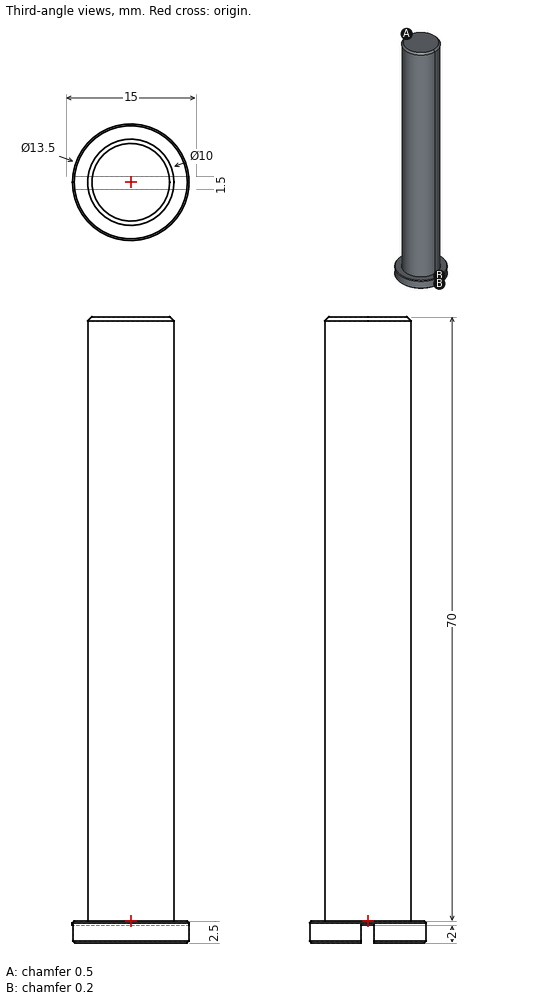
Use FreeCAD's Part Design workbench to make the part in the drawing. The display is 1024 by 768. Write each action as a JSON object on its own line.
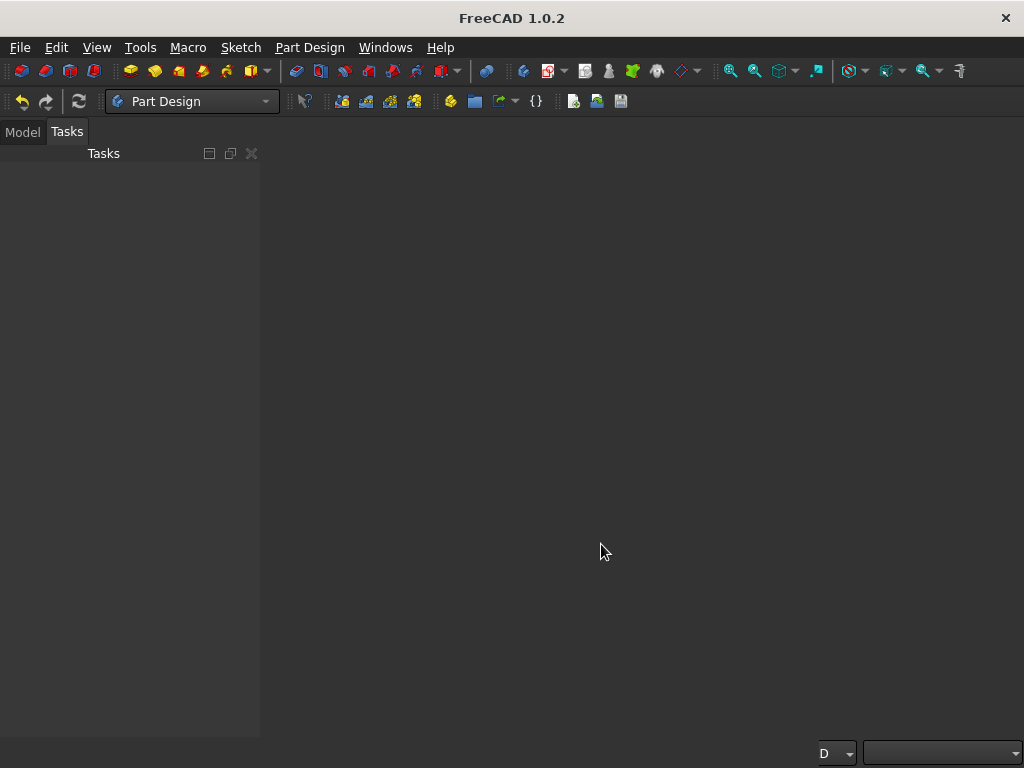
{"action": "left_click", "coordinate": [574, 102]}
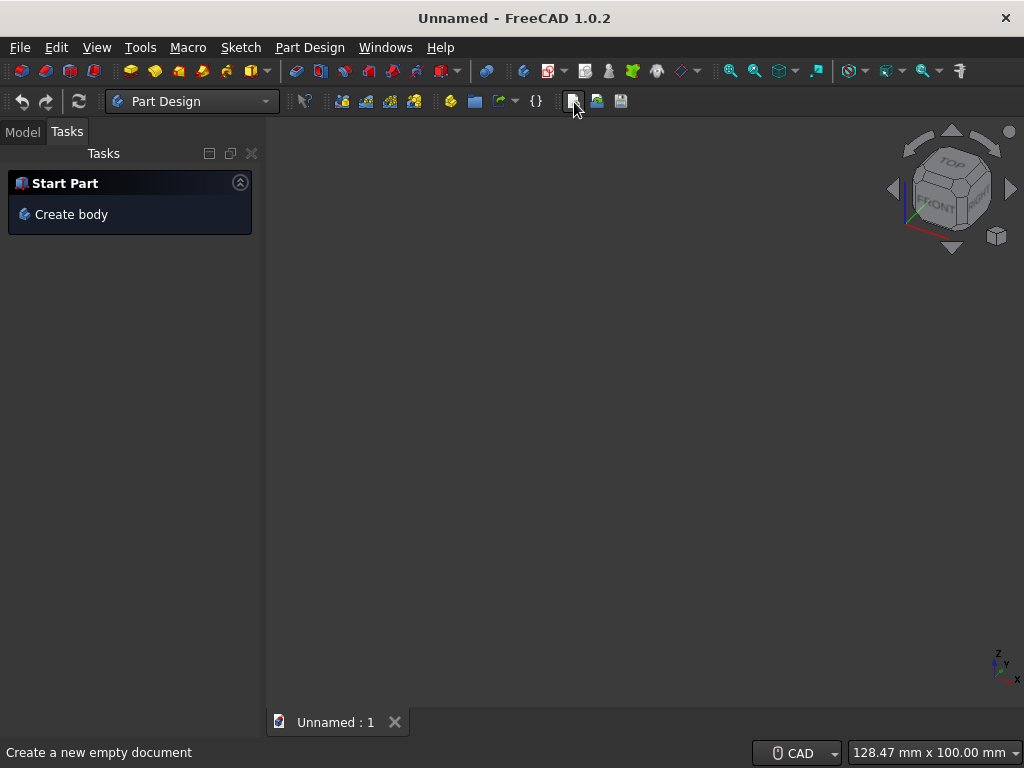
{"action": "left_click", "coordinate": [548, 72]}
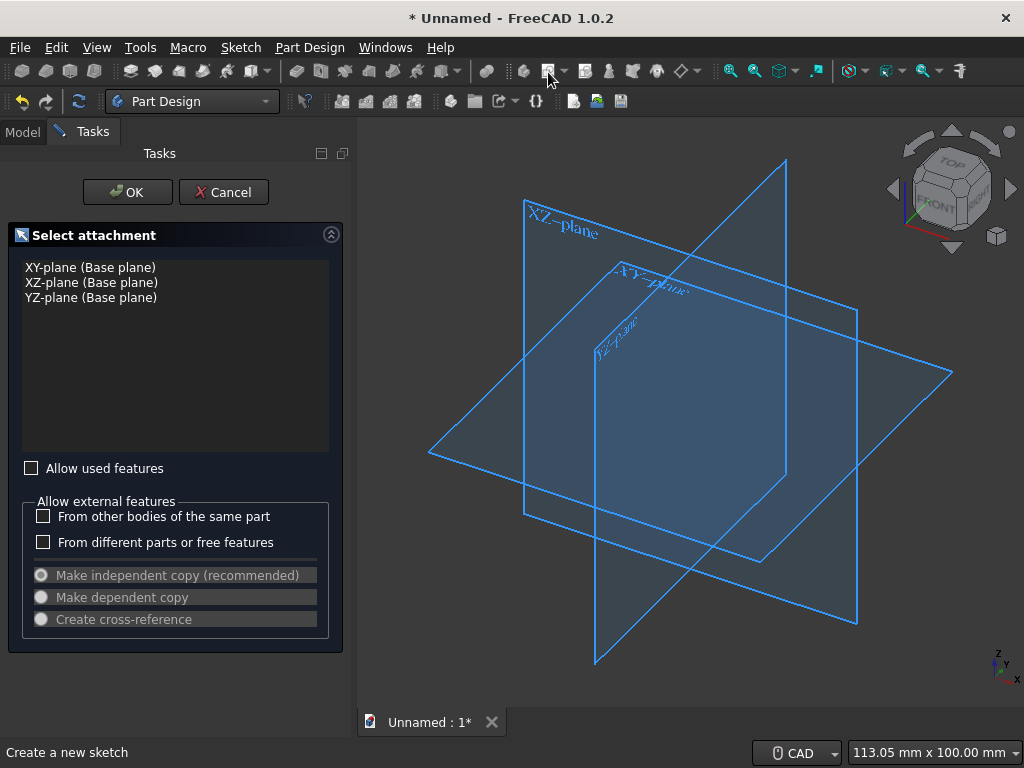
{"action": "left_click", "coordinate": [82, 268]}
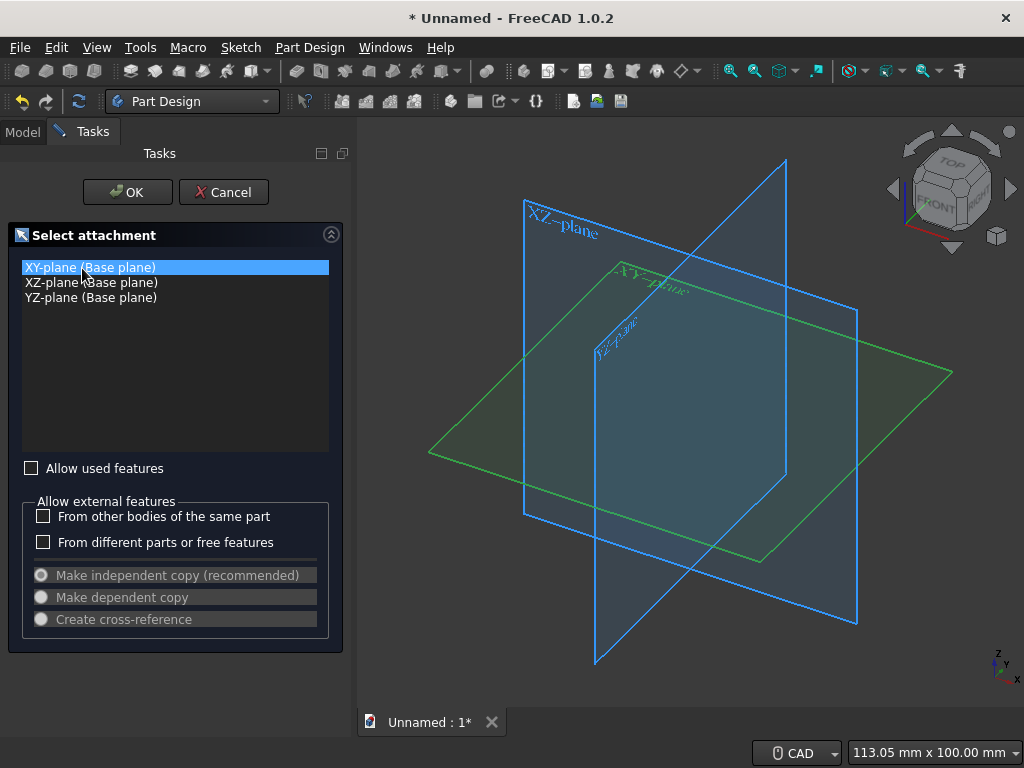
{"action": "left_click", "coordinate": [128, 192]}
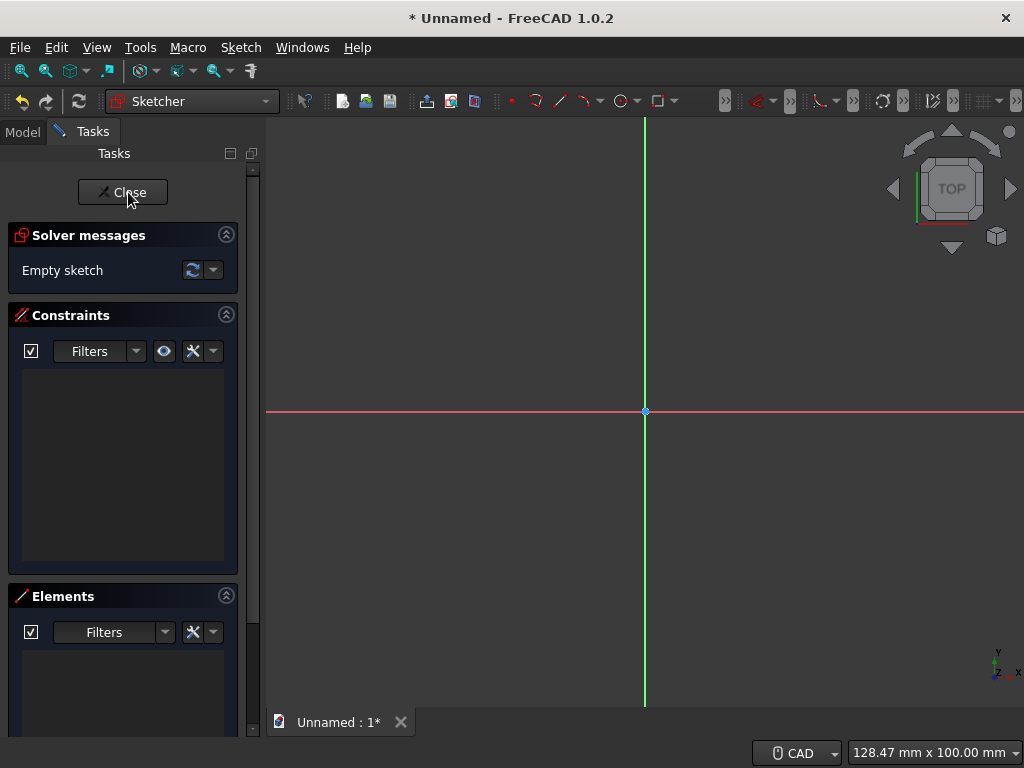
{"action": "scroll", "coordinate": [659, 412], "scroll_direction": "up", "scroll_amount": 9}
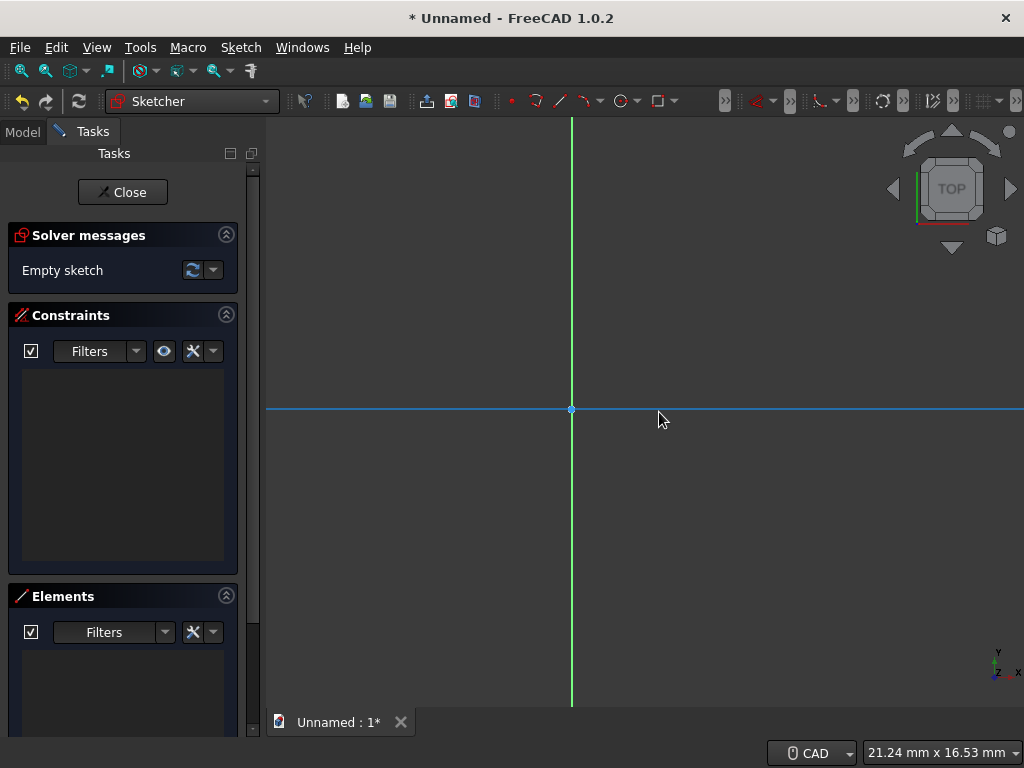
{"action": "key", "text": "g c"}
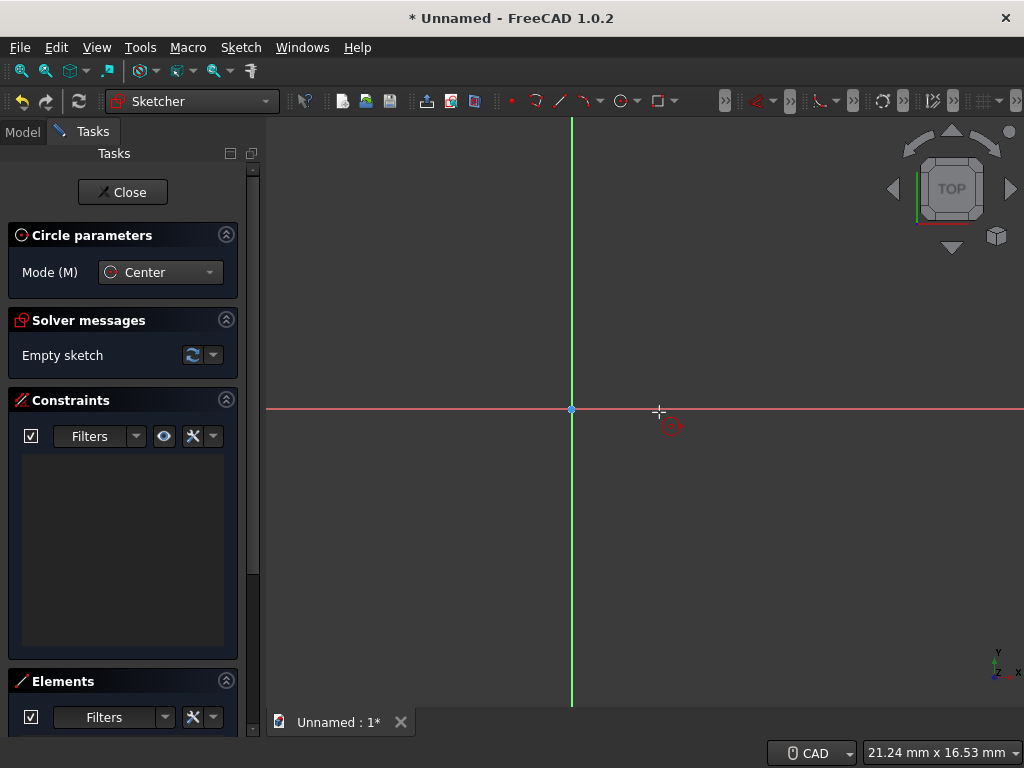
{"action": "left_click", "coordinate": [572, 409]}
{"action": "left_click", "coordinate": [698, 283]}
{"action": "key", "text": "Escape"}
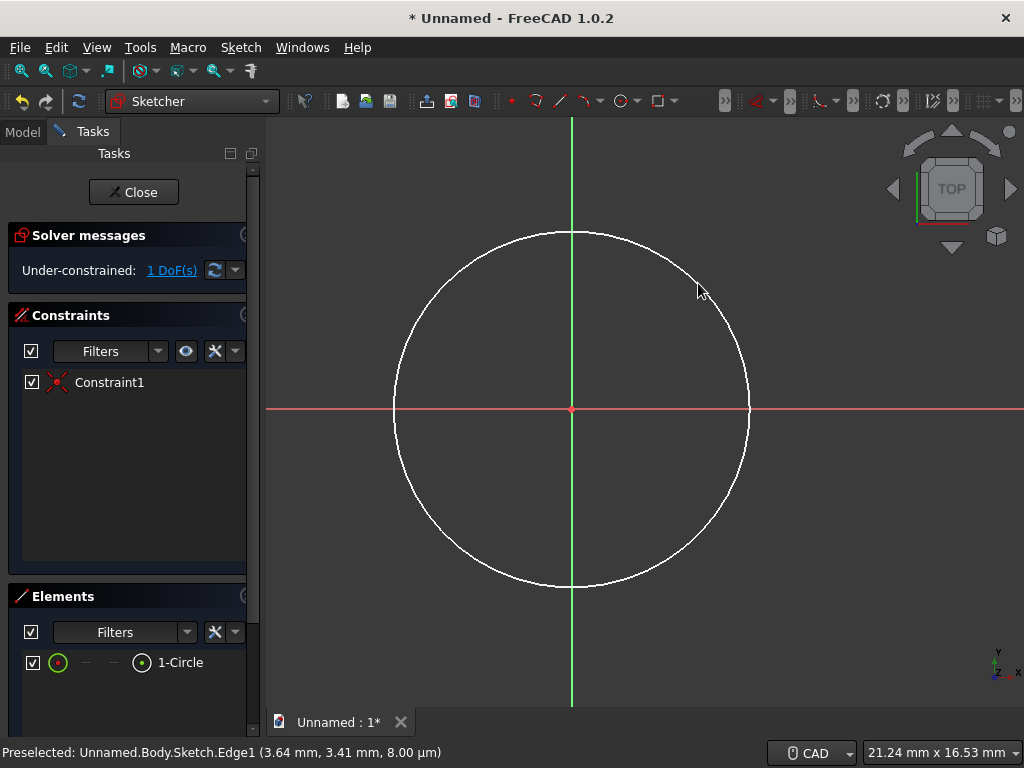
{"action": "left_click", "coordinate": [756, 102]}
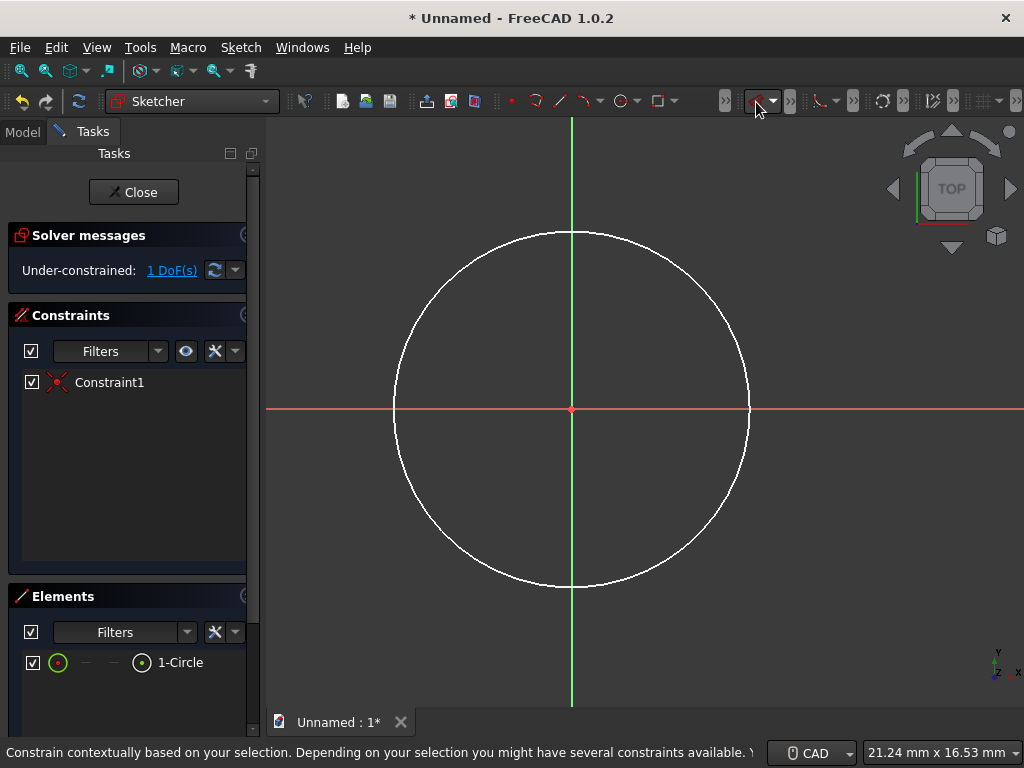
{"action": "left_click", "coordinate": [697, 283]}
{"action": "left_click", "coordinate": [720, 260]}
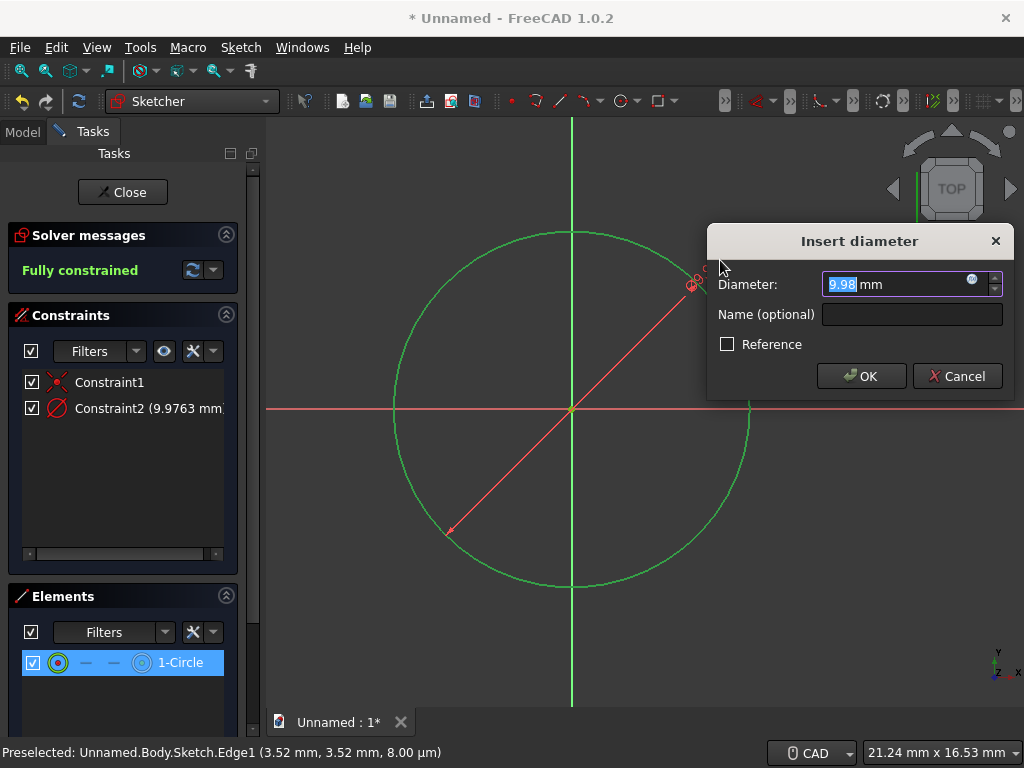
{"action": "type", "text": "10"}
{"action": "key", "text": "Return"}
{"action": "key", "text": "Escape"}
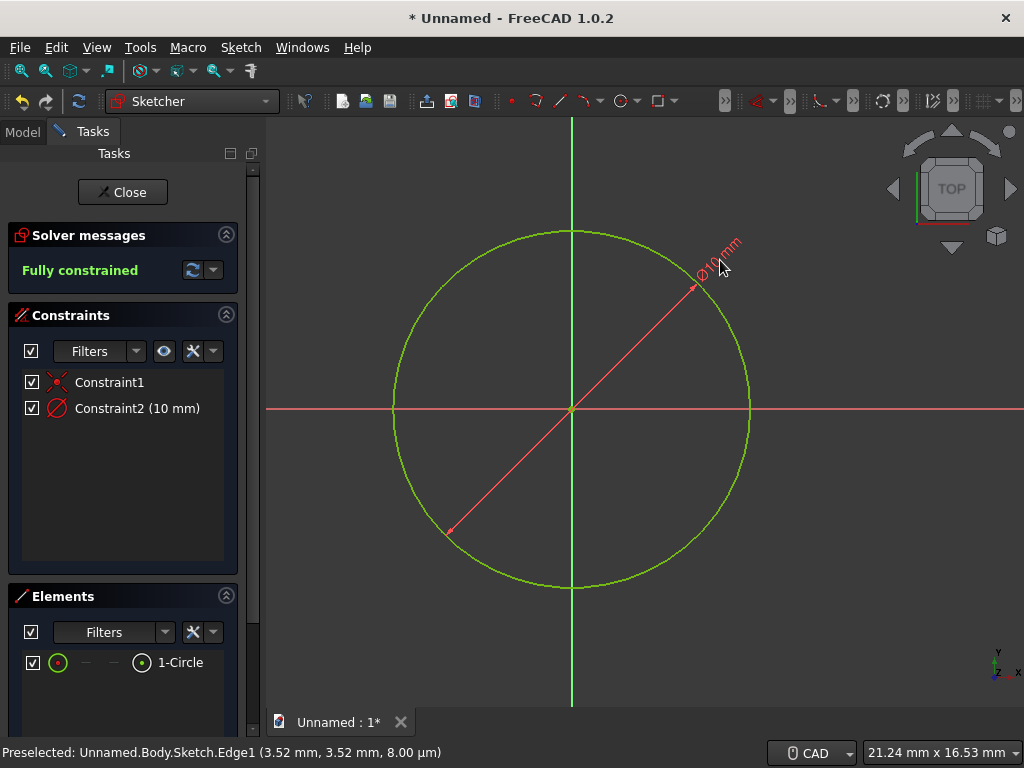
{"action": "left_click", "coordinate": [123, 192]}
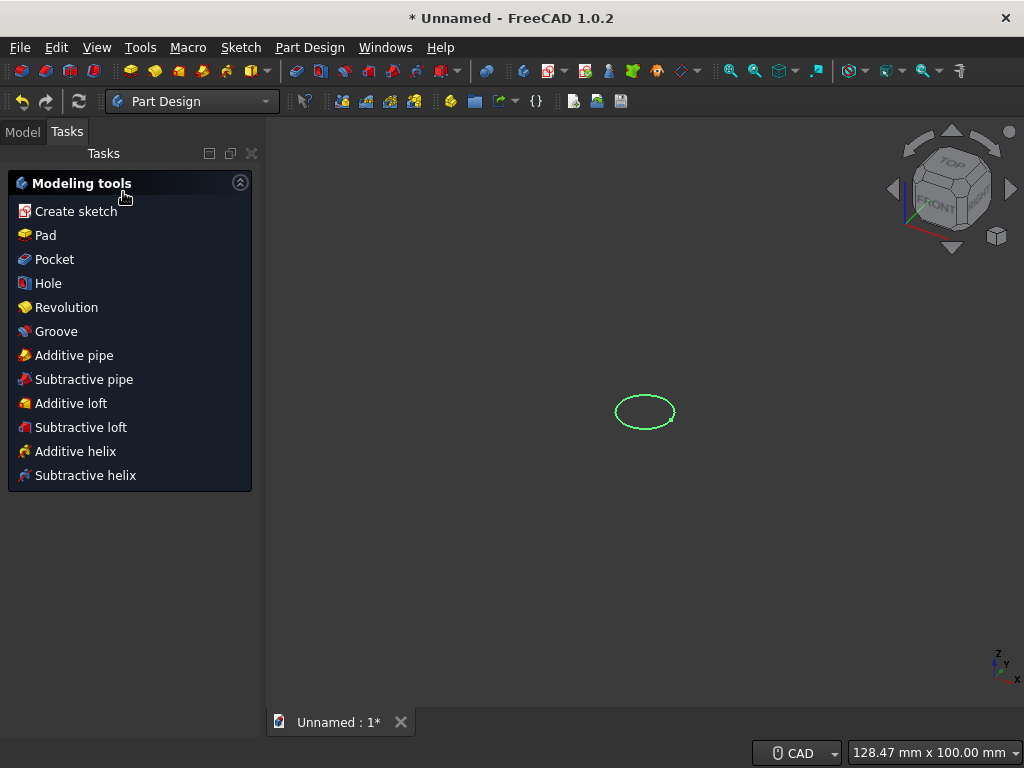
{"action": "left_click", "coordinate": [132, 72]}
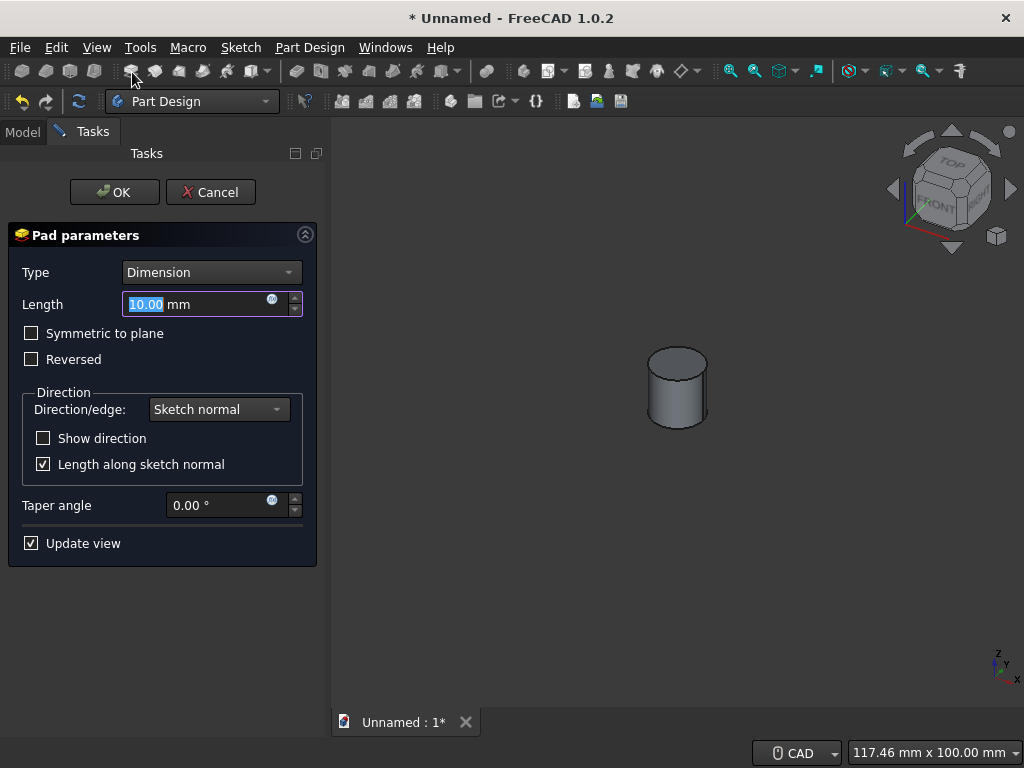
{"action": "type", "text": "70"}
{"action": "key", "text": "Tab"}